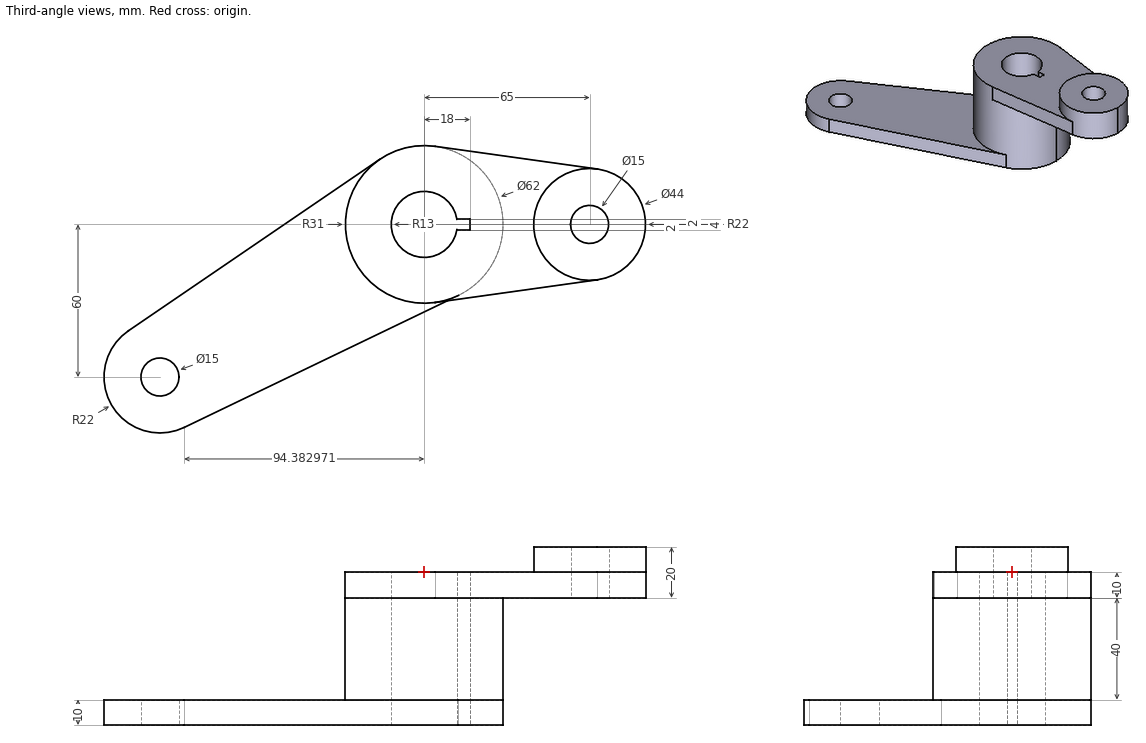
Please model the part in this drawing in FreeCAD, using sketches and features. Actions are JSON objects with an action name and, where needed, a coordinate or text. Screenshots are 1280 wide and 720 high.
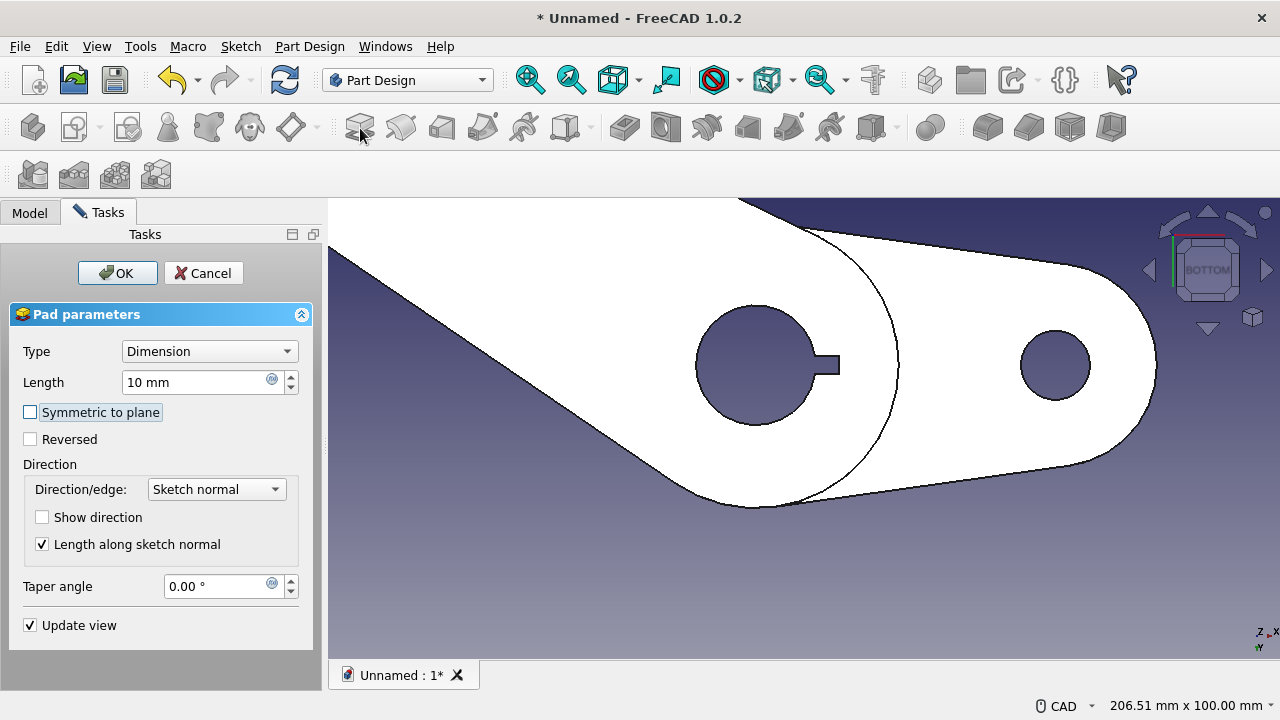
{"action": "left_click", "coordinate": [118, 273]}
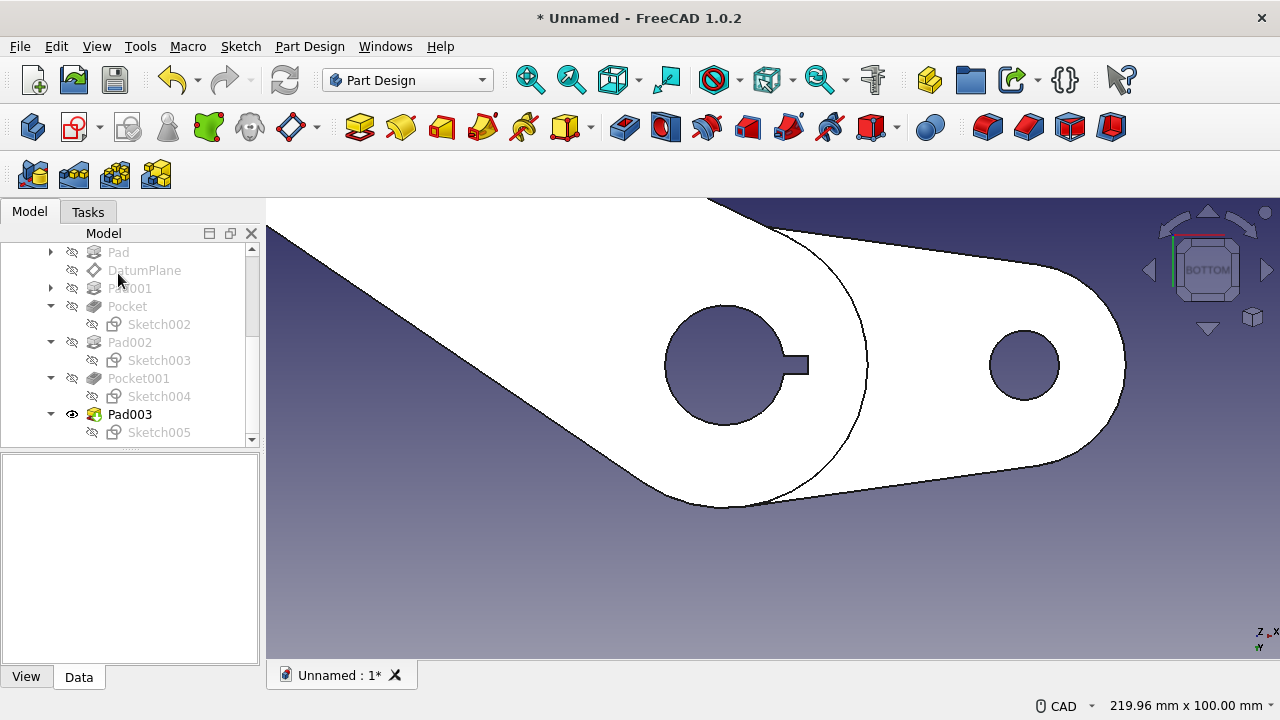
{"action": "key", "text": "0"}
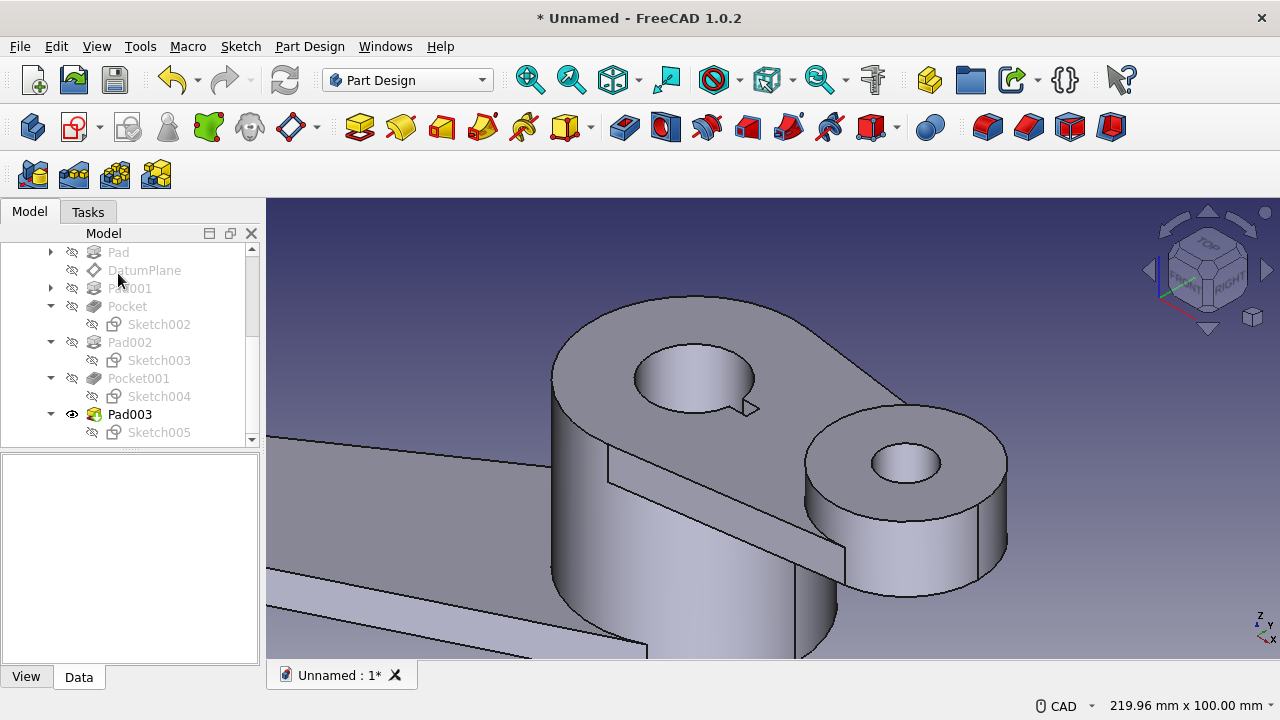
{"action": "left_click", "coordinate": [531, 80]}